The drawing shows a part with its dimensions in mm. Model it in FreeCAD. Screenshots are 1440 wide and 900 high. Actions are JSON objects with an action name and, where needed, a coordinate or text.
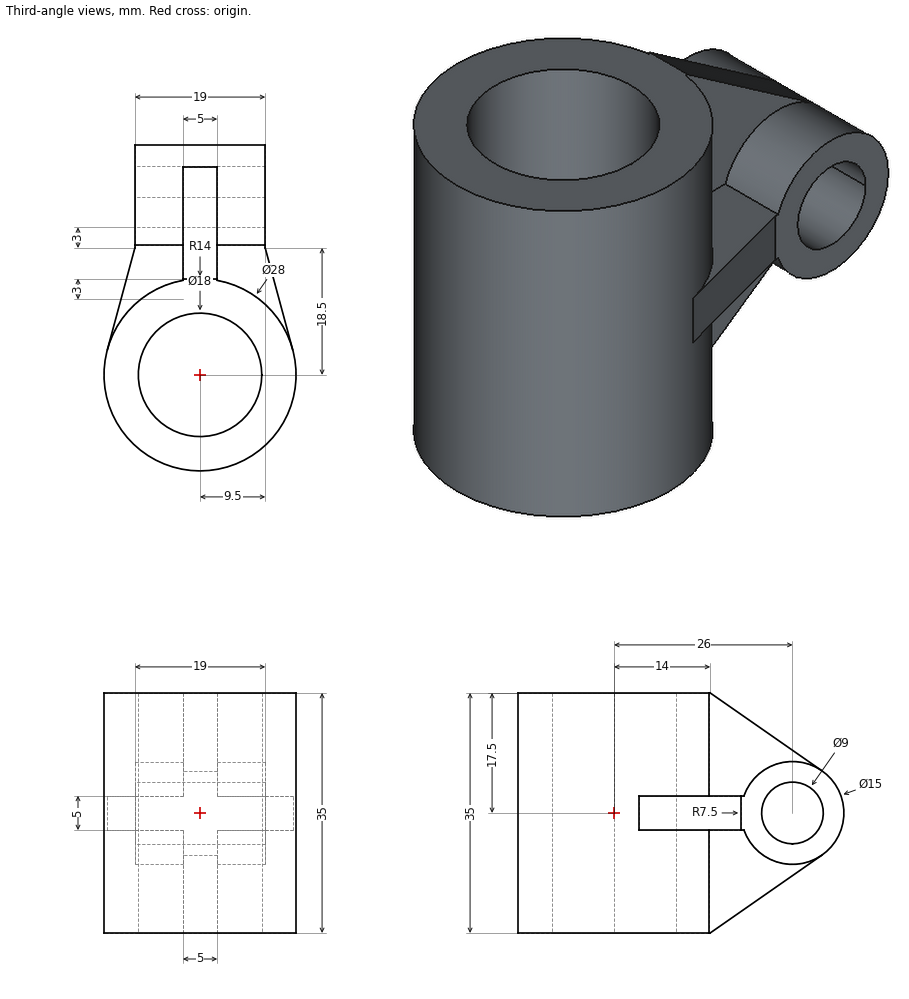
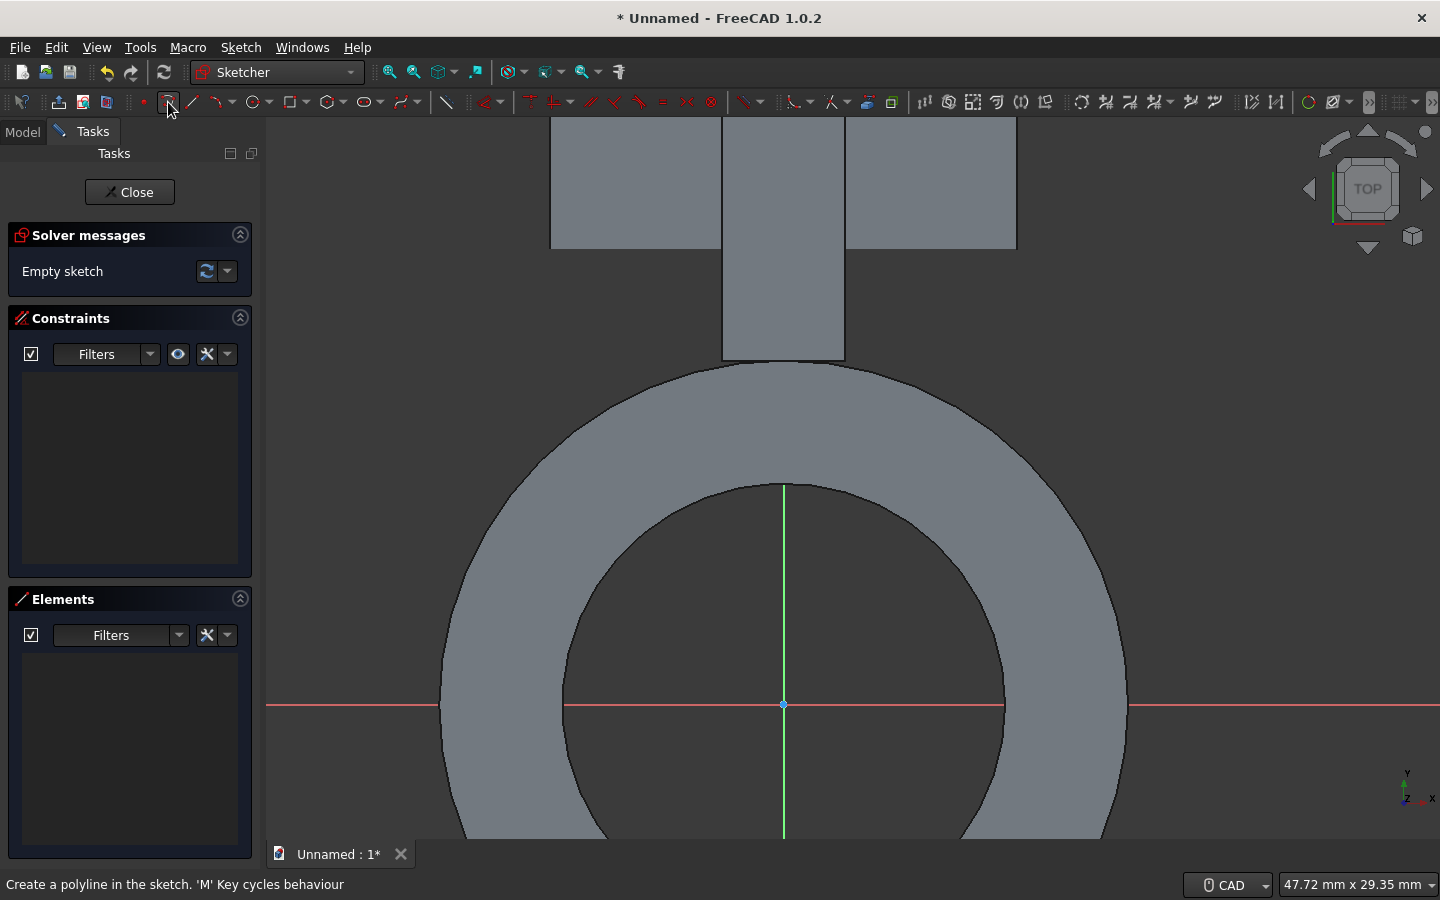
{"action": "left_click", "coordinate": [1116, 615]}
{"action": "left_click", "coordinate": [1017, 250]}
{"action": "left_click", "coordinate": [550, 250]}
{"action": "left_click", "coordinate": [451, 615]}
{"action": "right_click", "coordinate": [451, 615]}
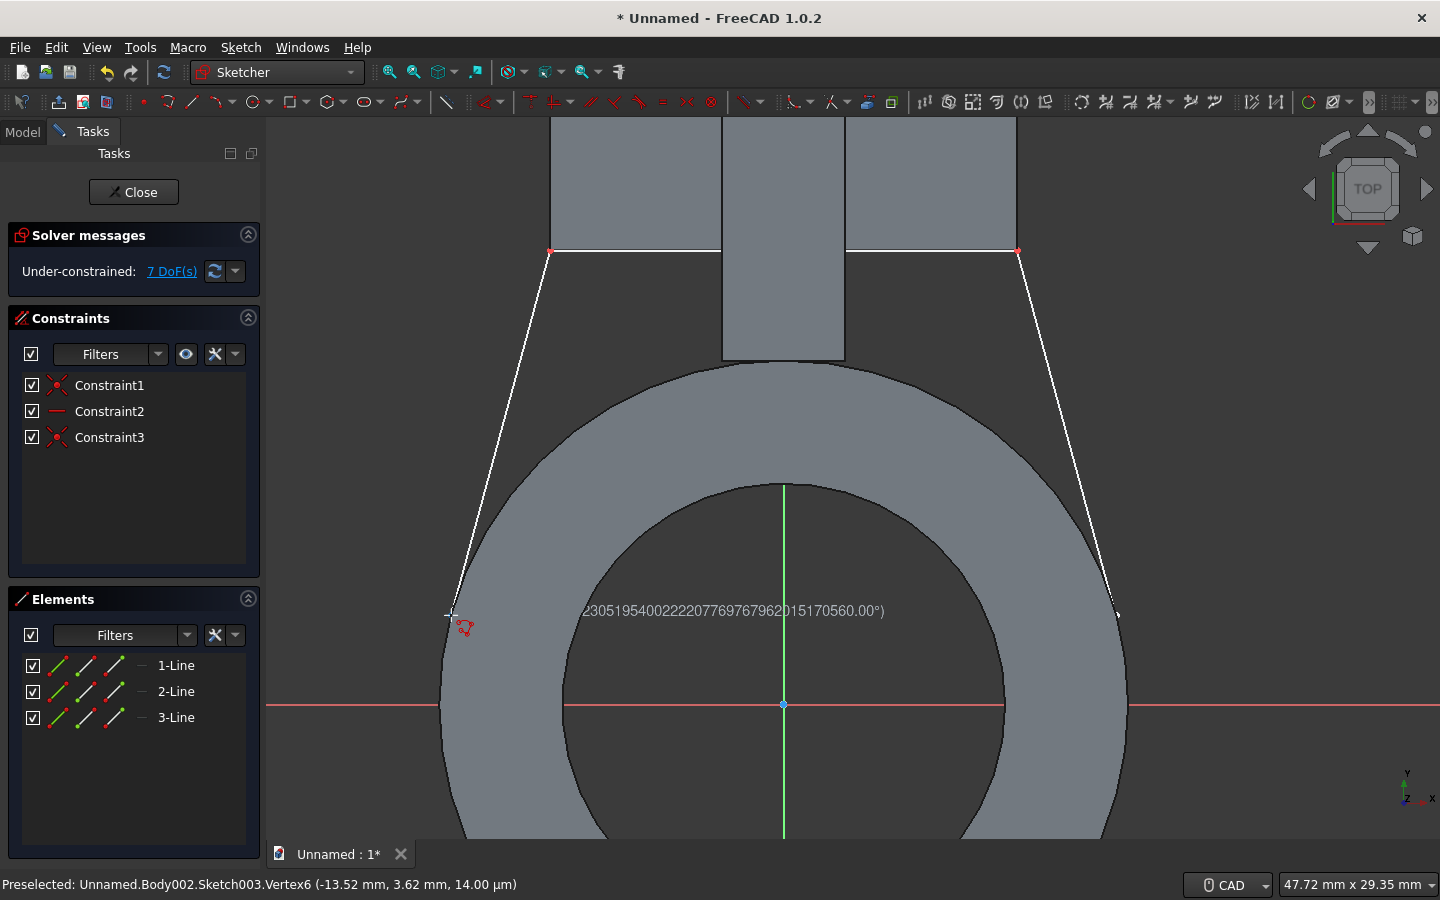
{"action": "key", "text": "g 3 a"}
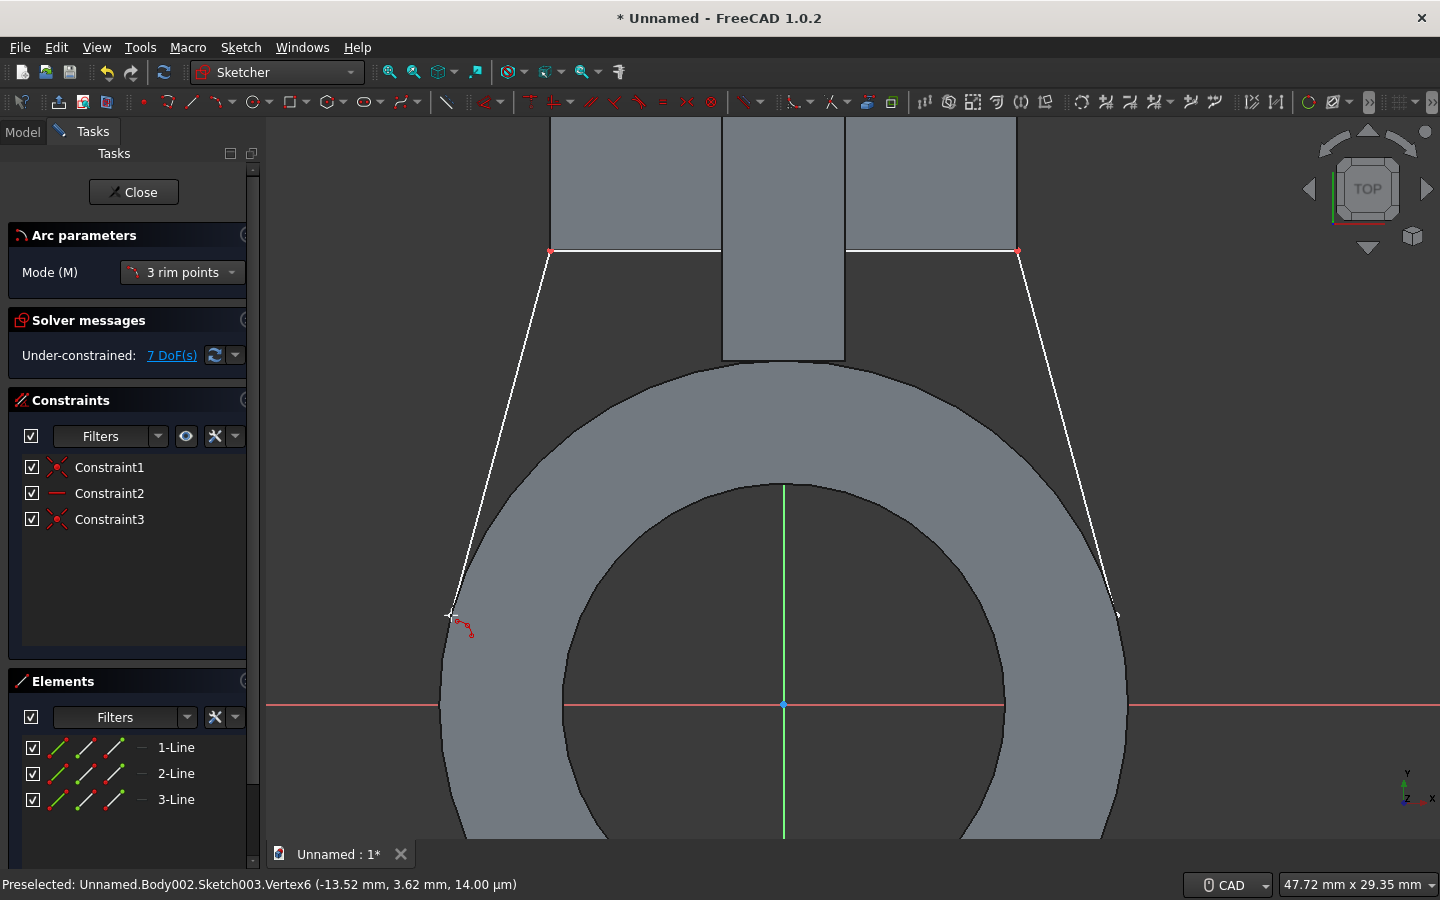
{"action": "left_click", "coordinate": [451, 616]}
{"action": "left_click", "coordinate": [1116, 616]}
{"action": "left_click", "coordinate": [873, 372]}
{"action": "key", "text": "Escape"}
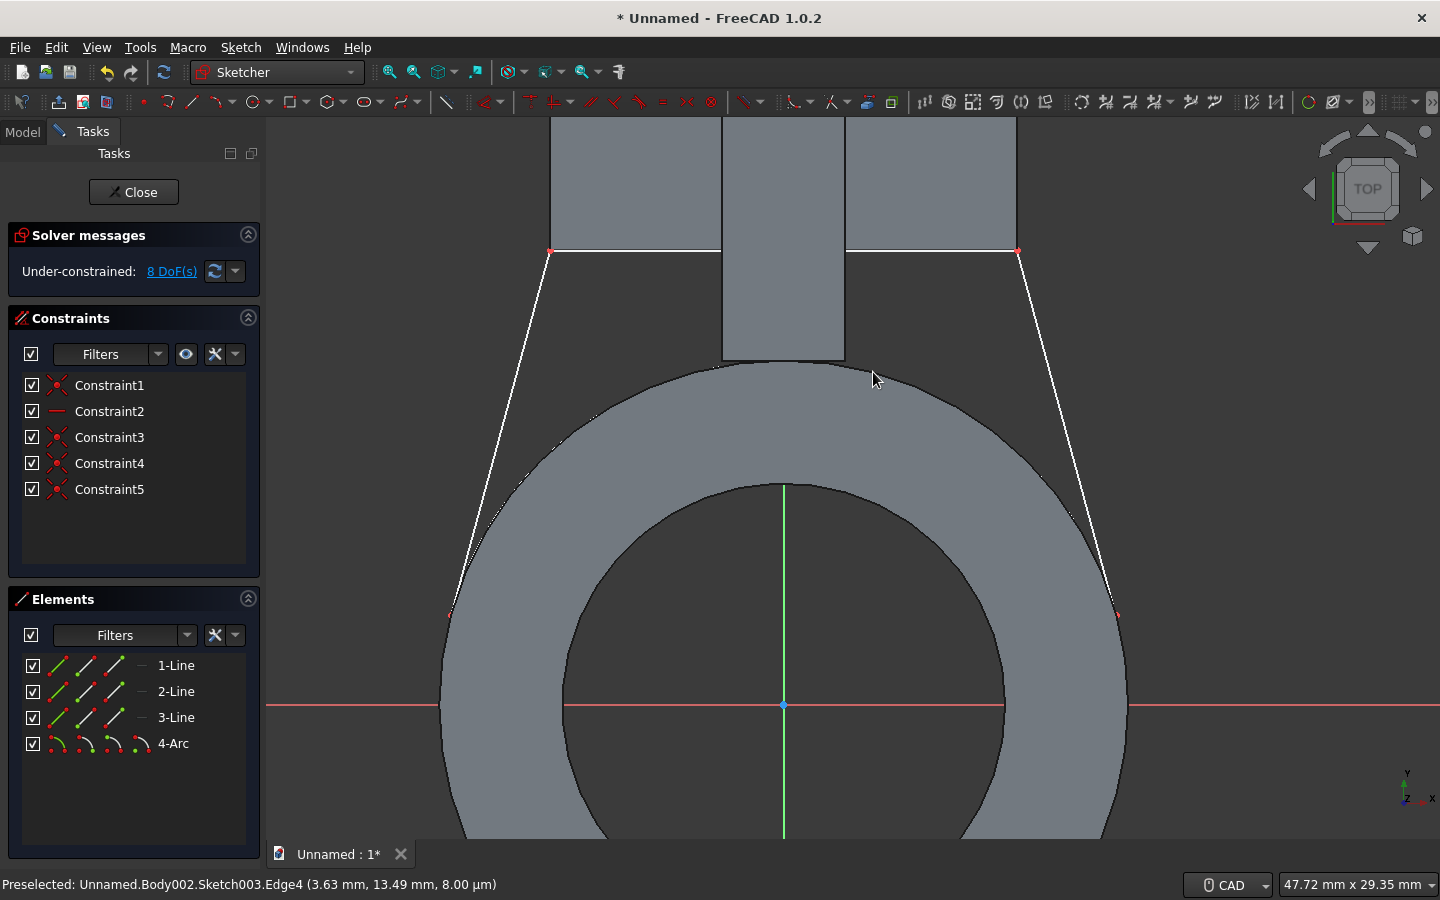
{"action": "left_click", "coordinate": [1086, 506]}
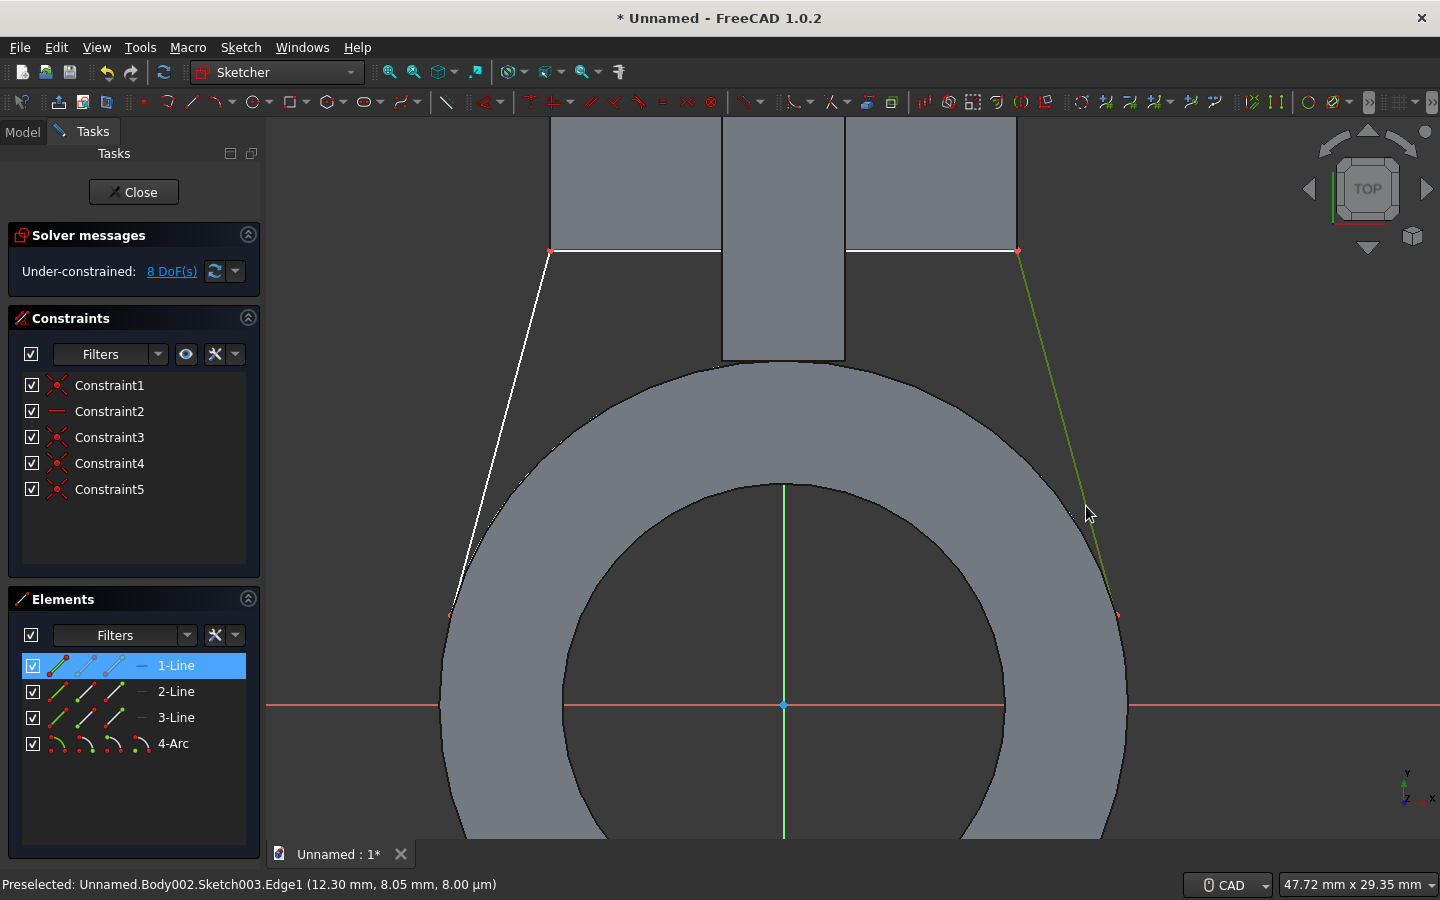
{"action": "left_click", "coordinate": [956, 407]}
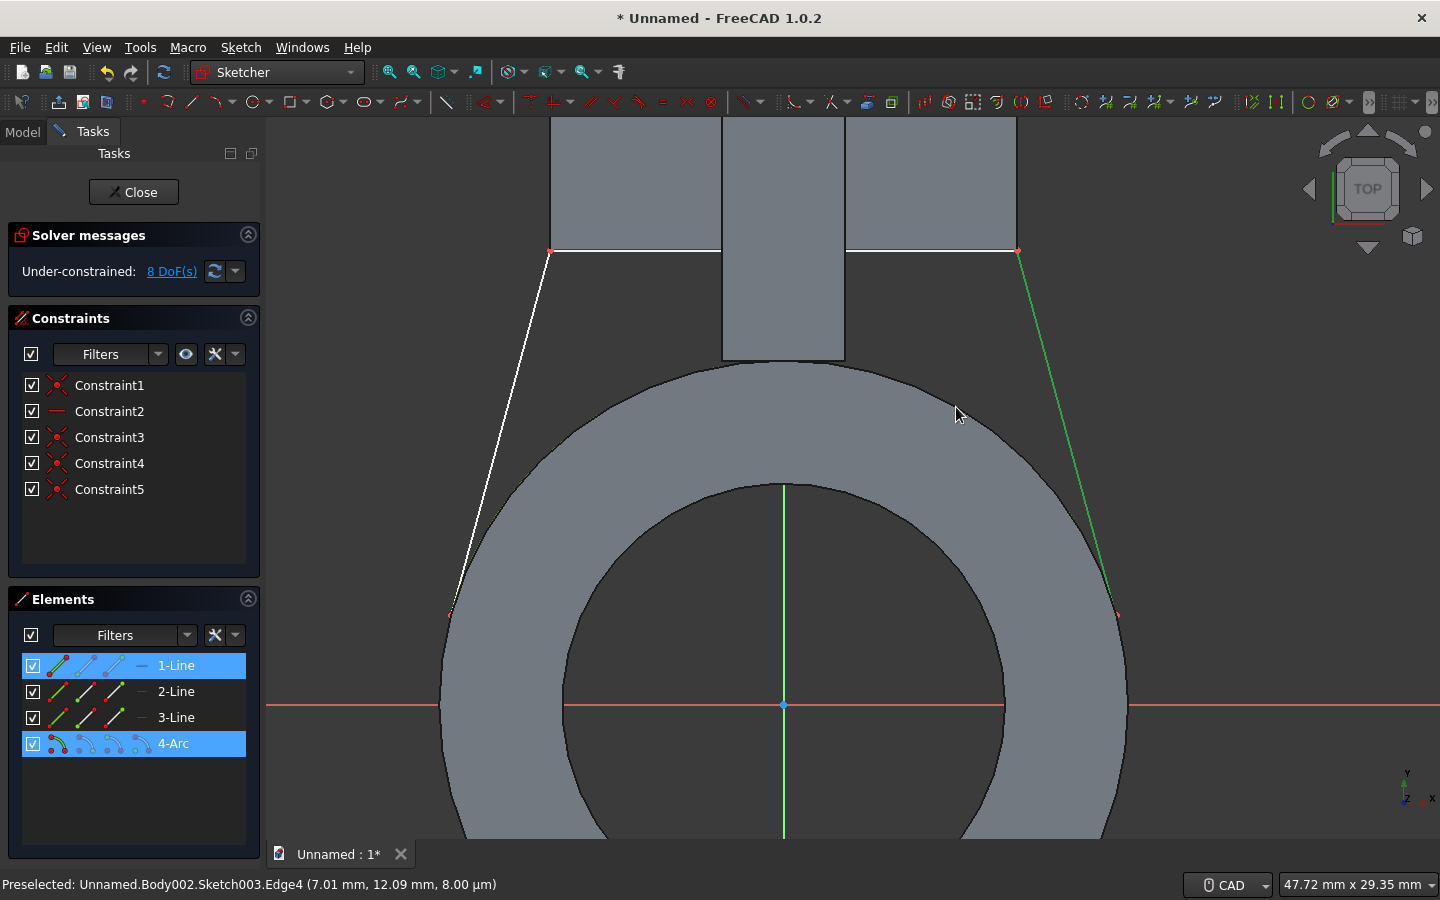
{"action": "key", "text": "t"}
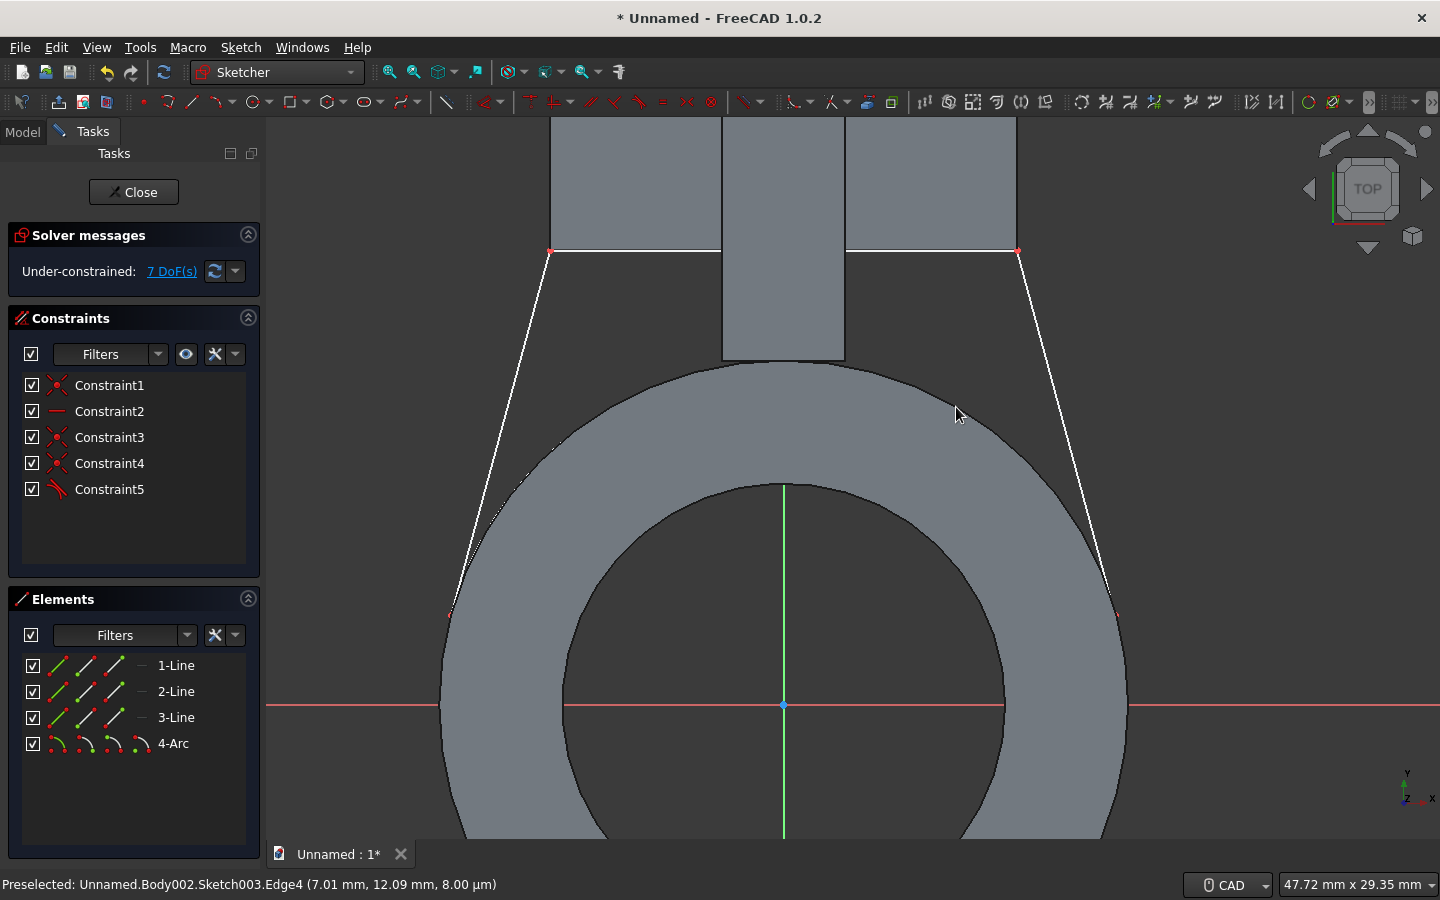
{"action": "left_click", "coordinate": [520, 361]}